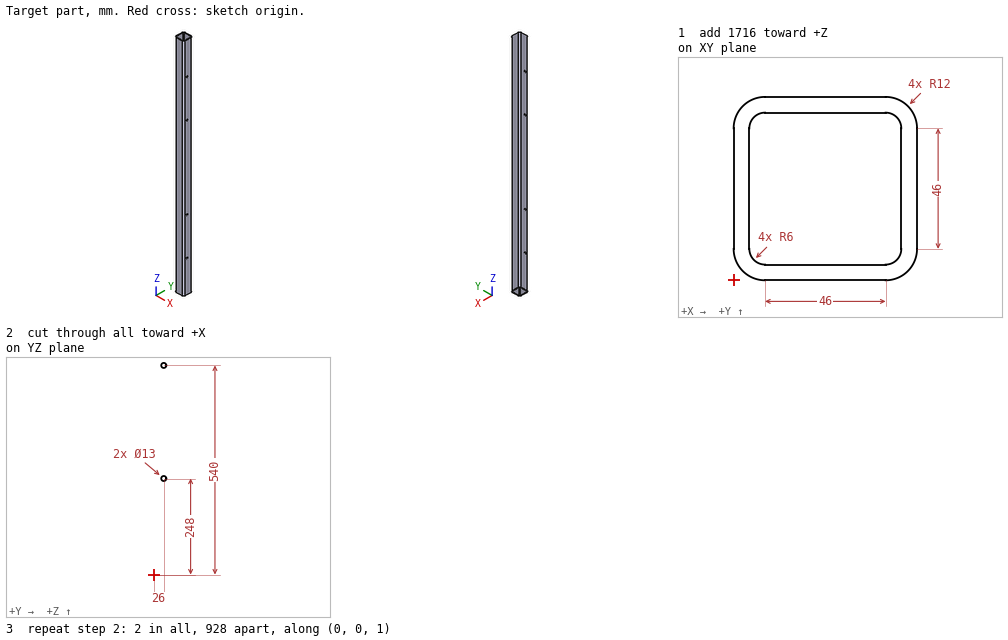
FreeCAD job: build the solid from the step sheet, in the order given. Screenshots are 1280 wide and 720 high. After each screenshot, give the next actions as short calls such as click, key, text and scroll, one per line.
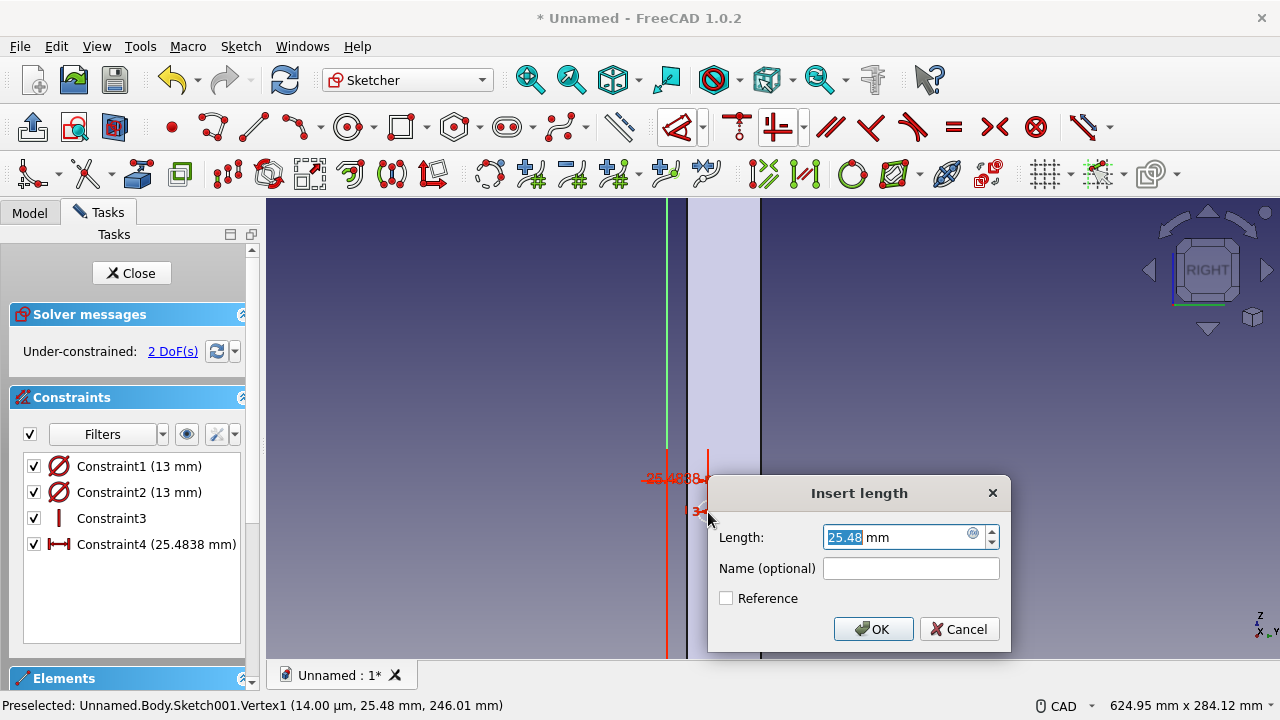
text(26)
key(Return)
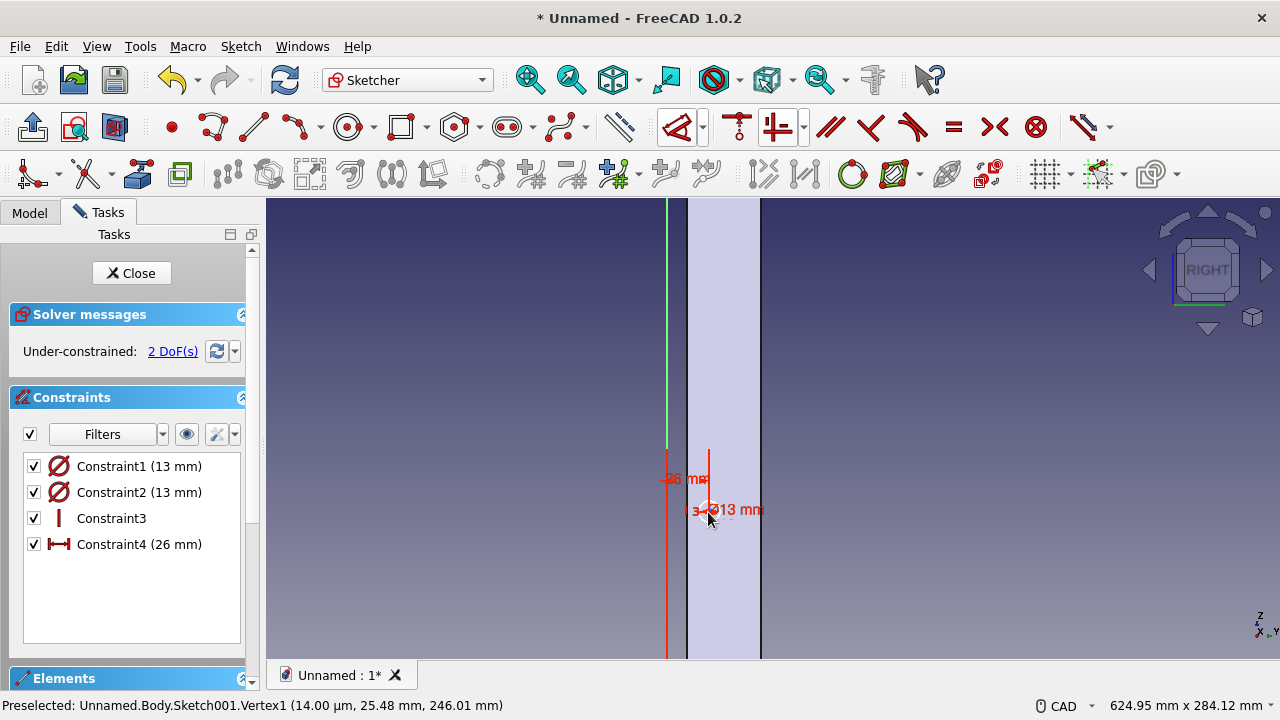
click(709, 512)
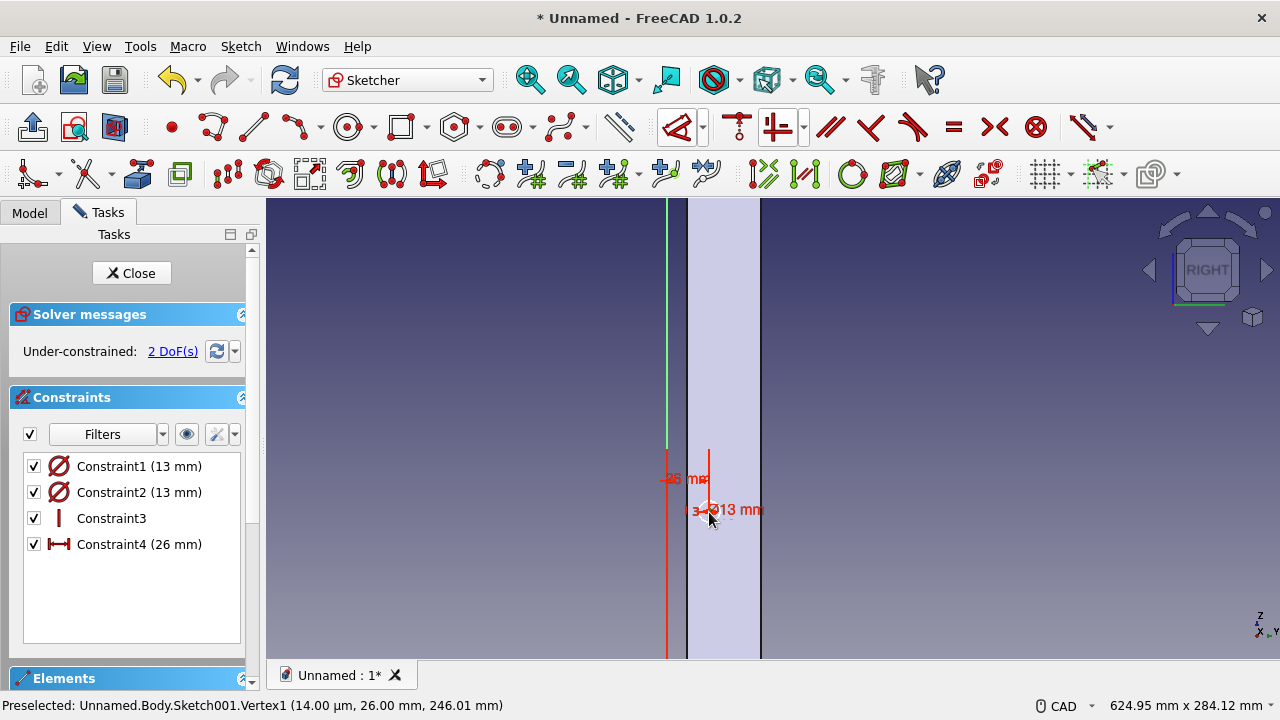
key(i)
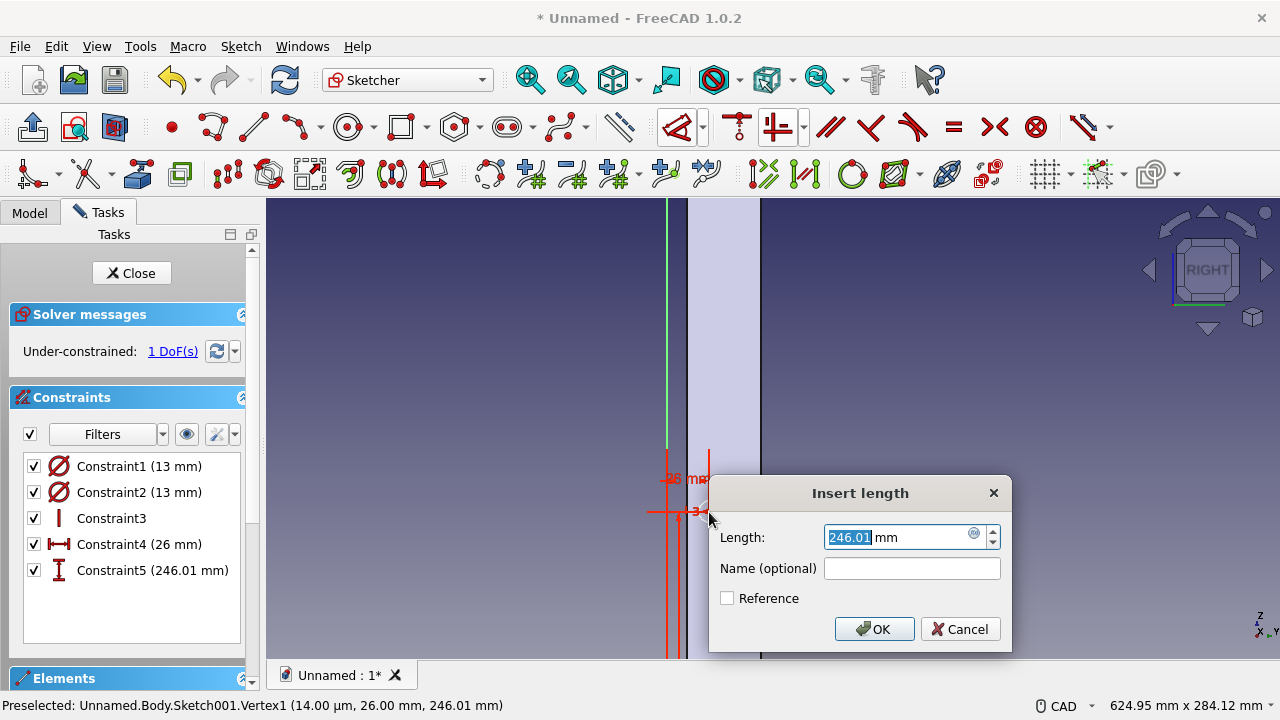
text(248)
key(Return)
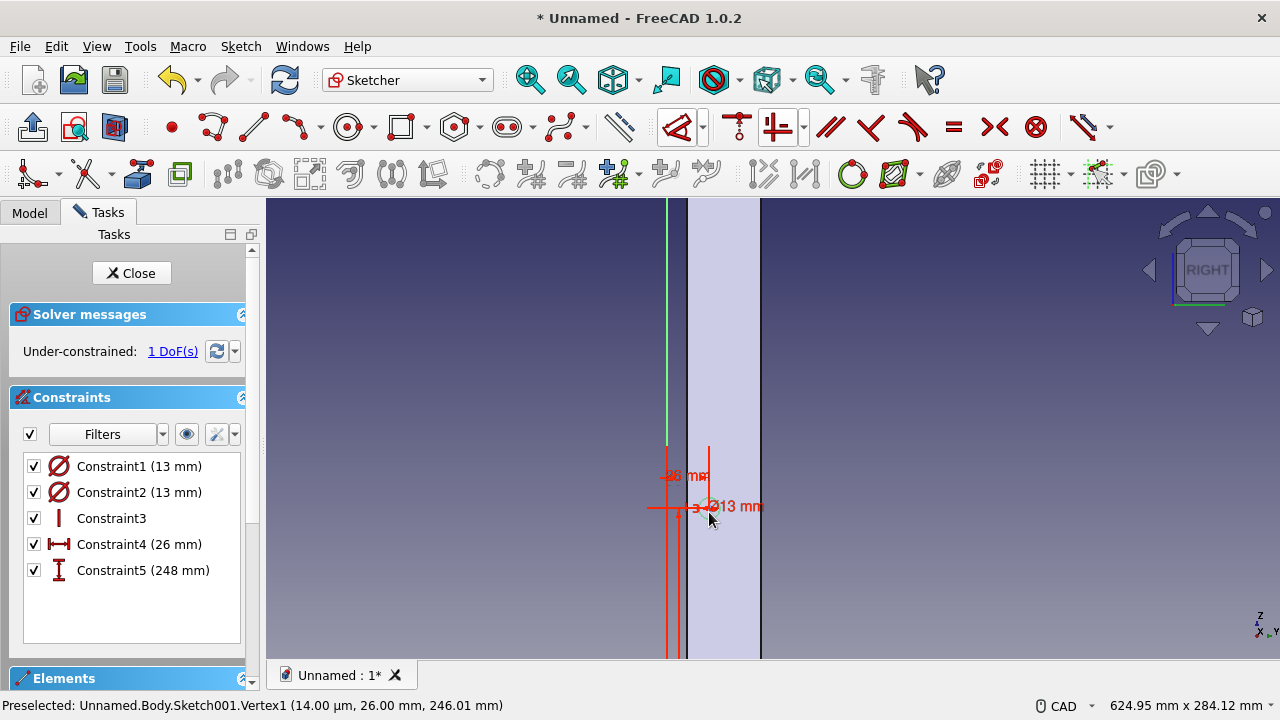
scroll(709, 412, down, 6)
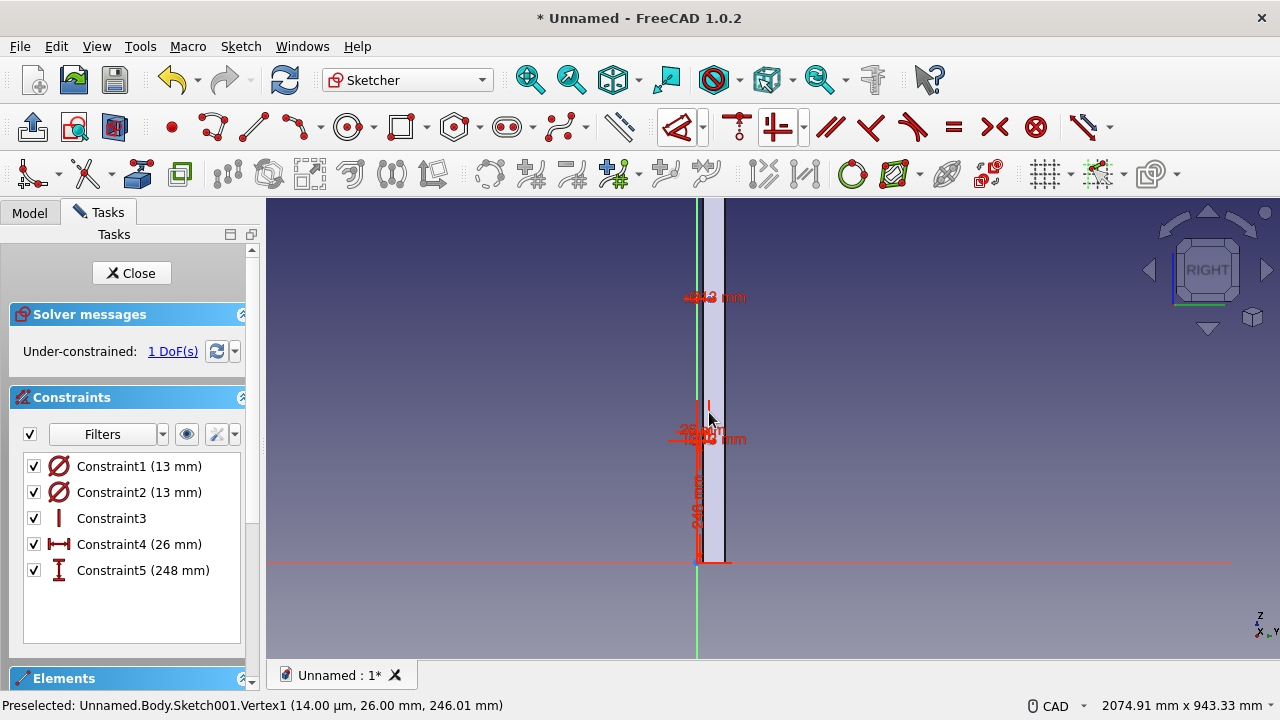
click(709, 299)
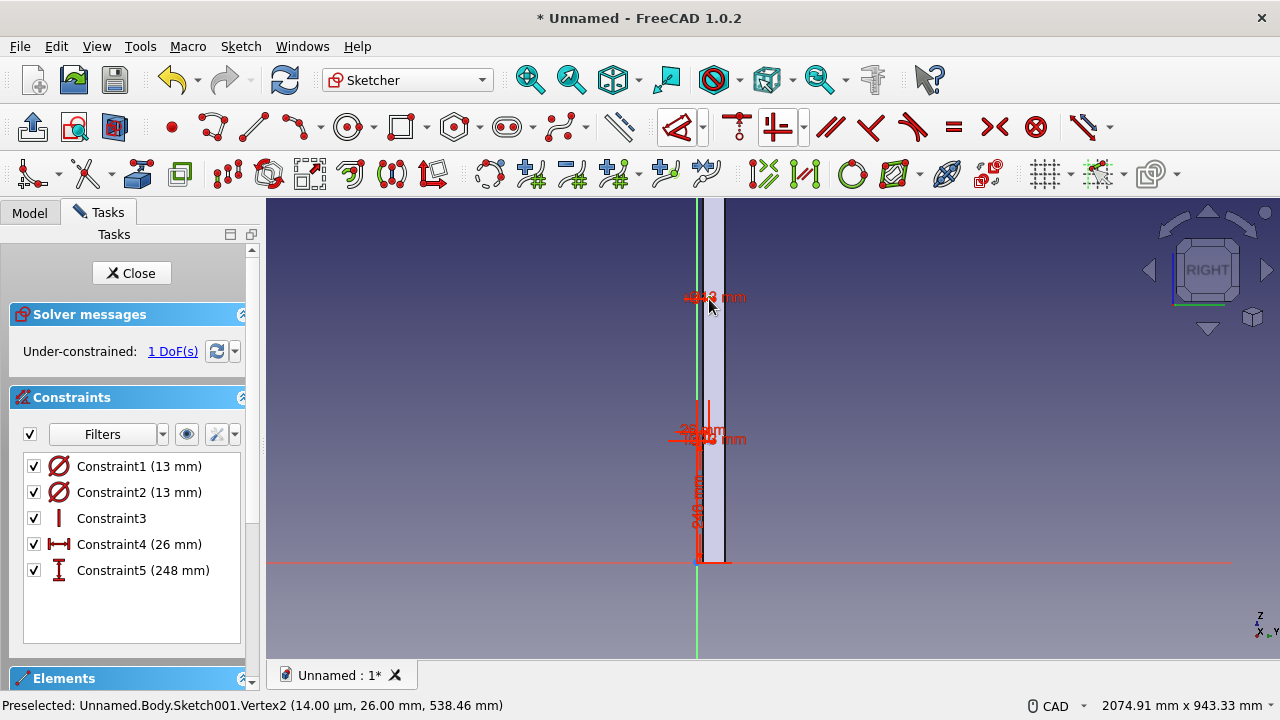
click(702, 128)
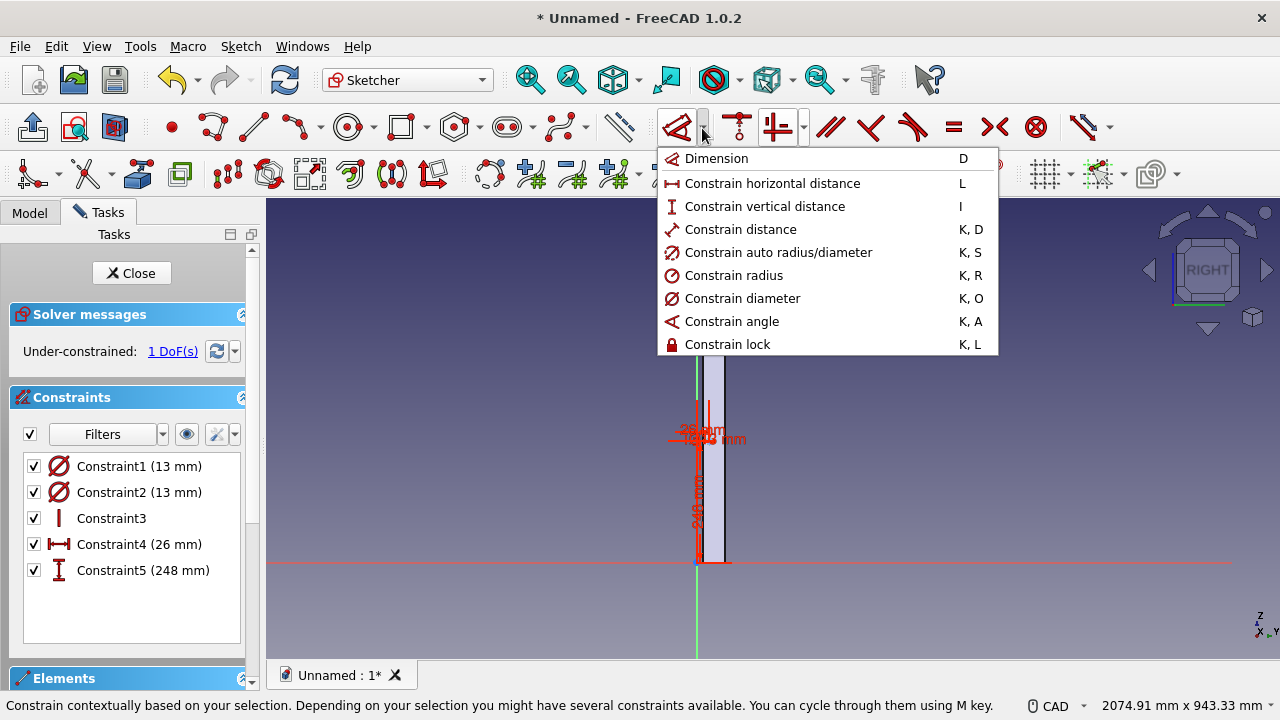
click(828, 206)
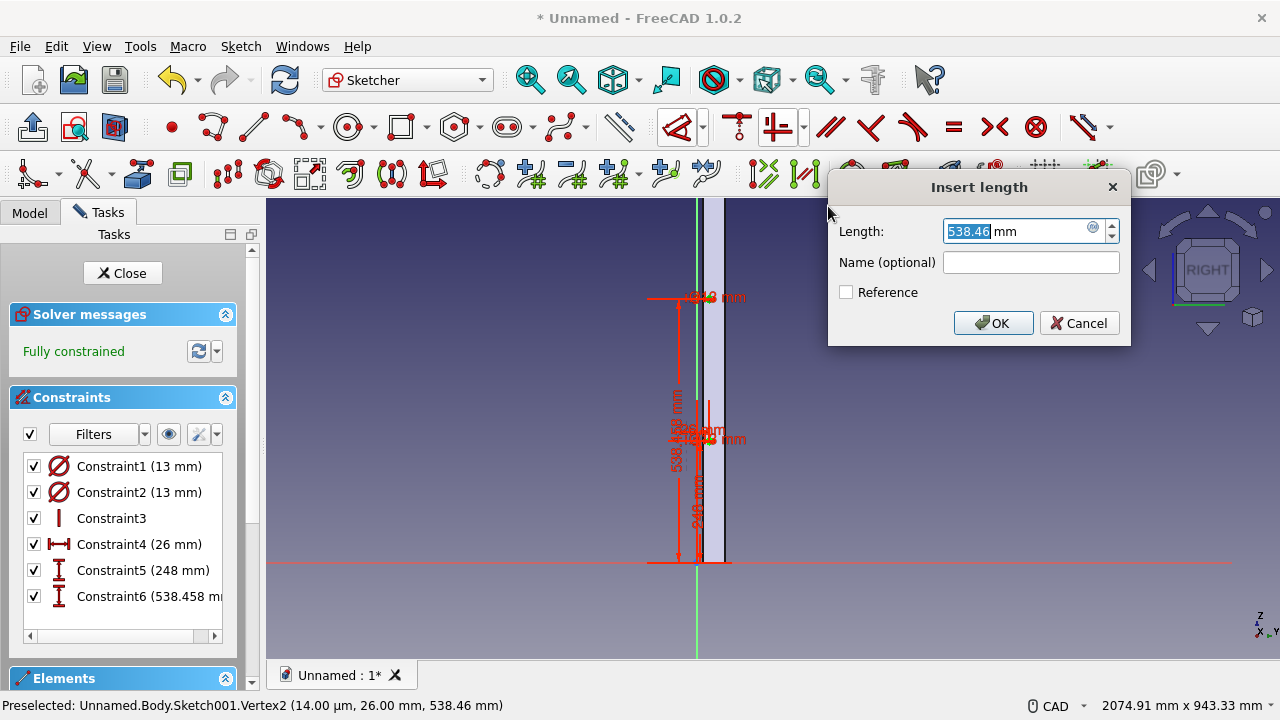
text(540)
key(Return)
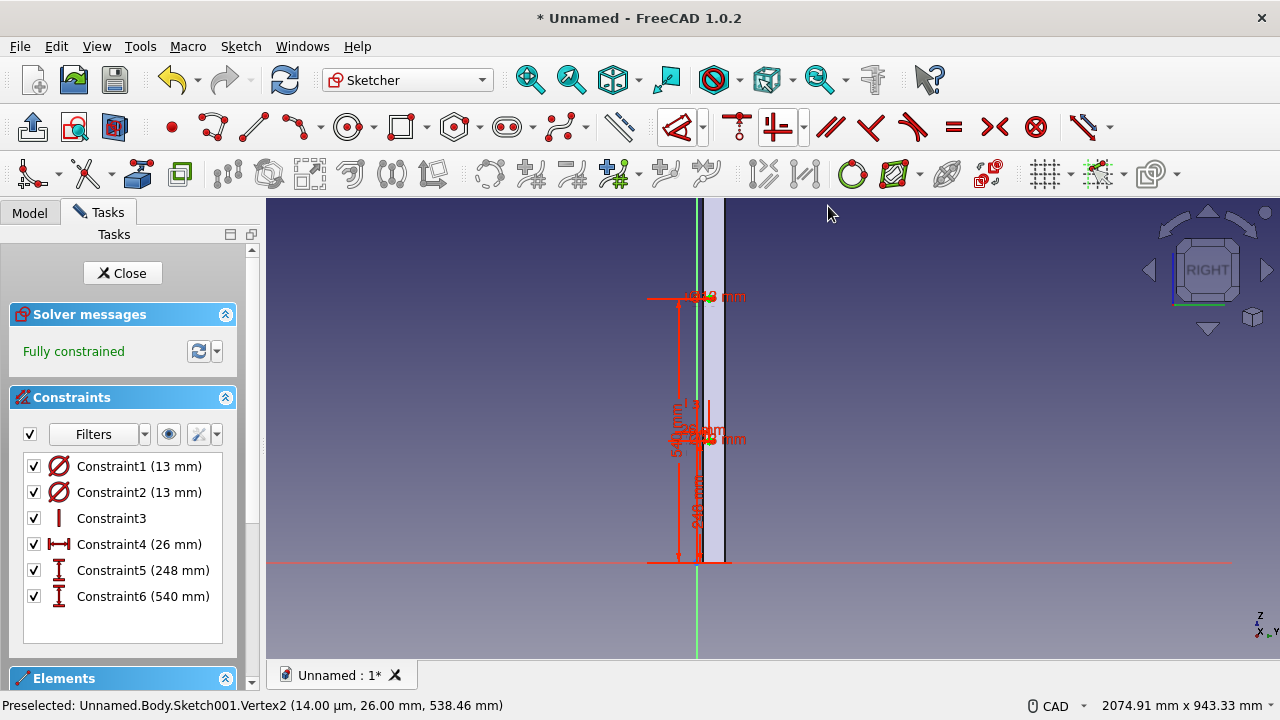
click(123, 273)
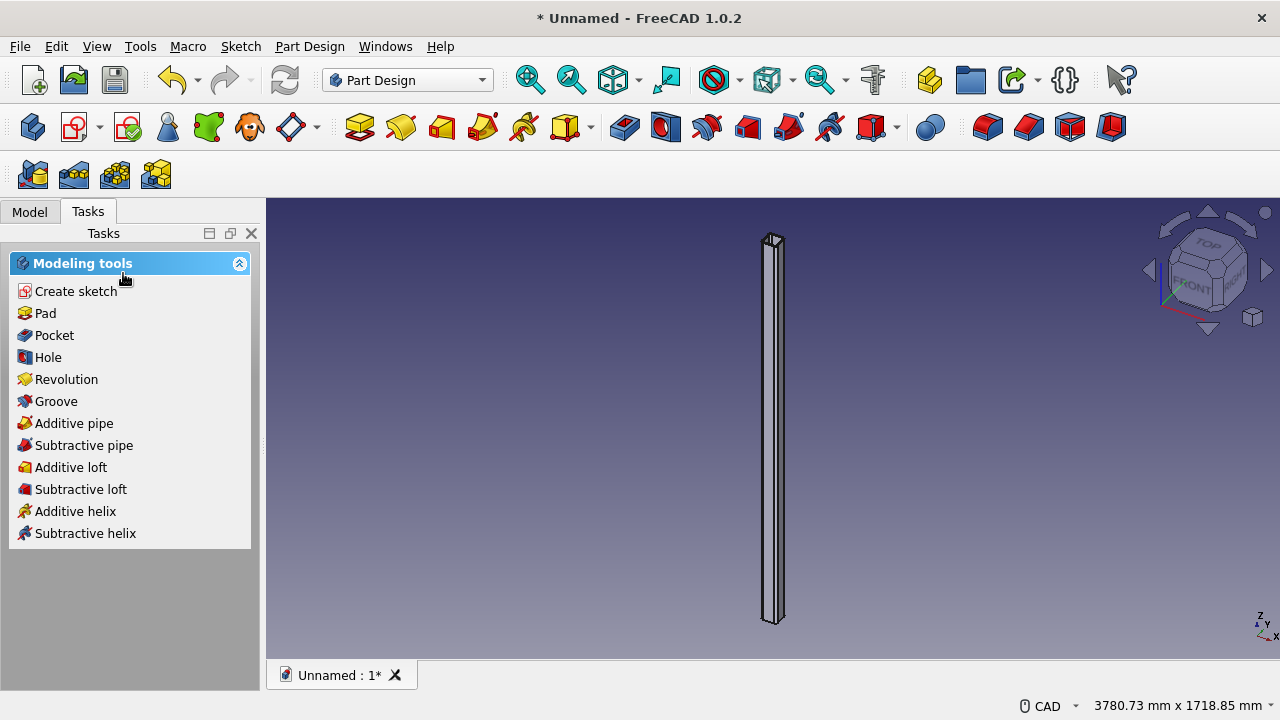
click(625, 128)